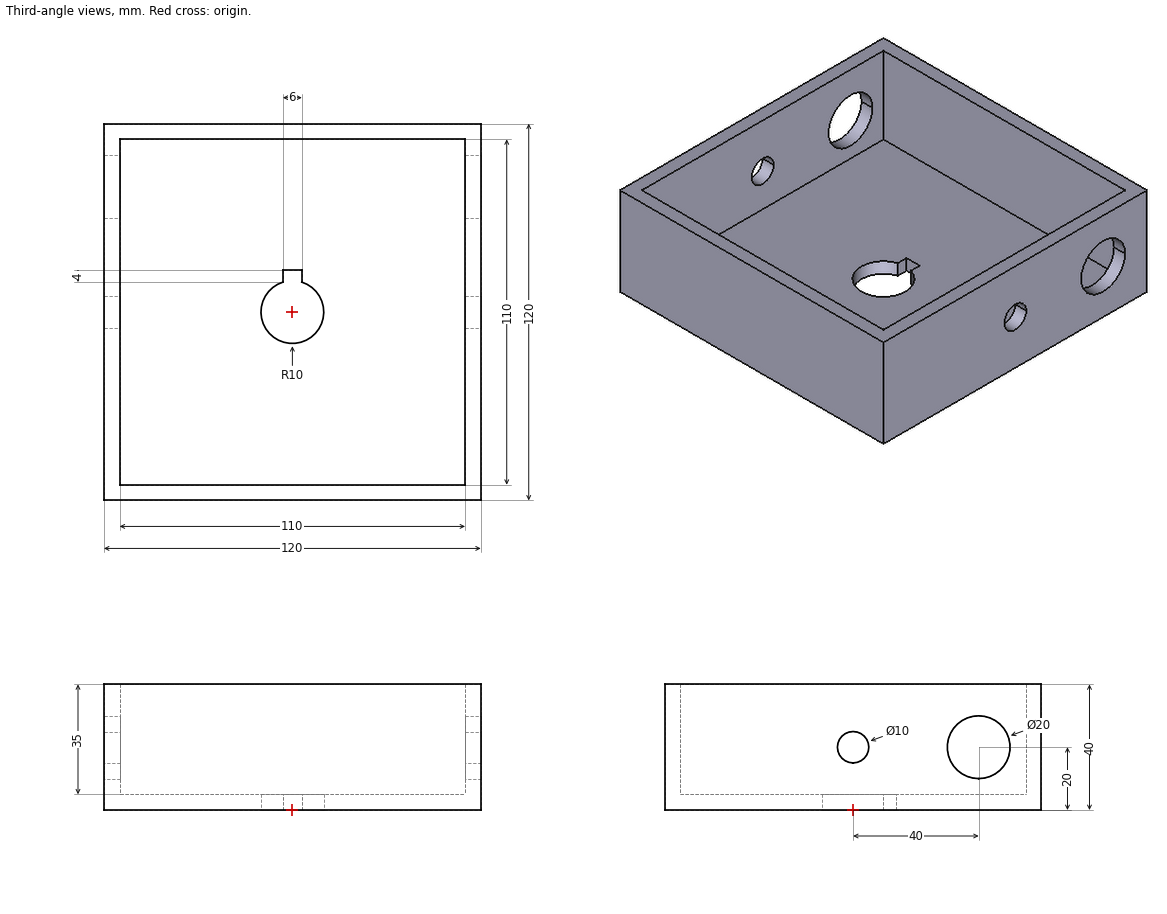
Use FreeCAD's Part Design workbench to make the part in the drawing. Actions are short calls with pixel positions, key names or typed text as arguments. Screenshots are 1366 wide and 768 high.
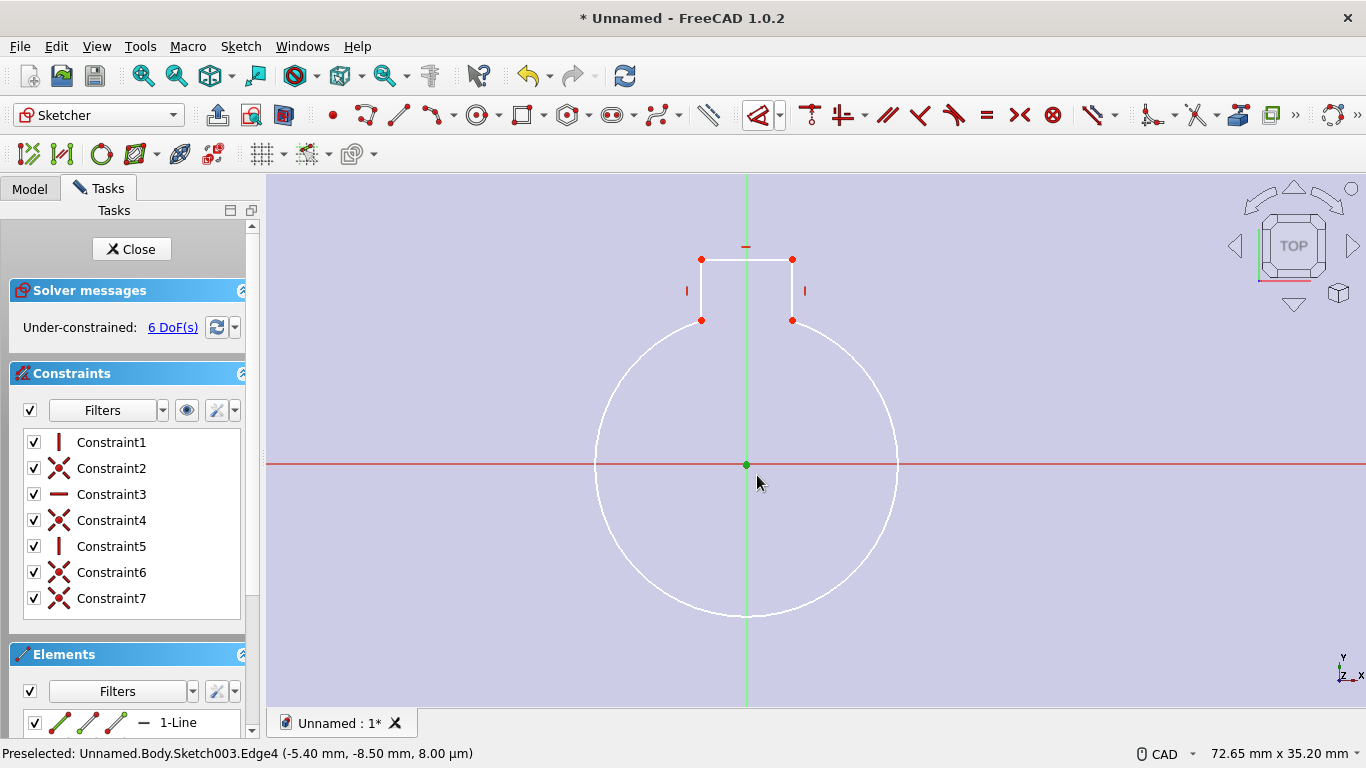
key(c)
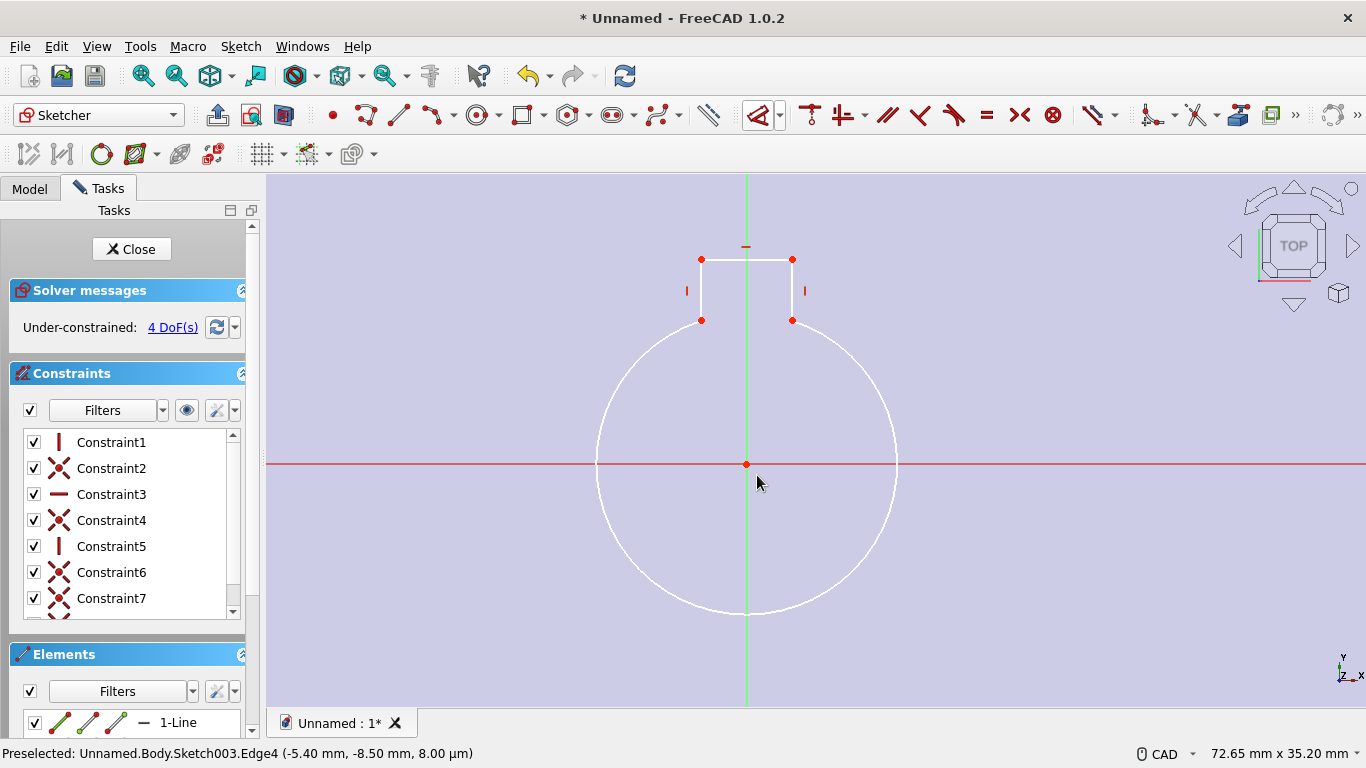
click(611, 528)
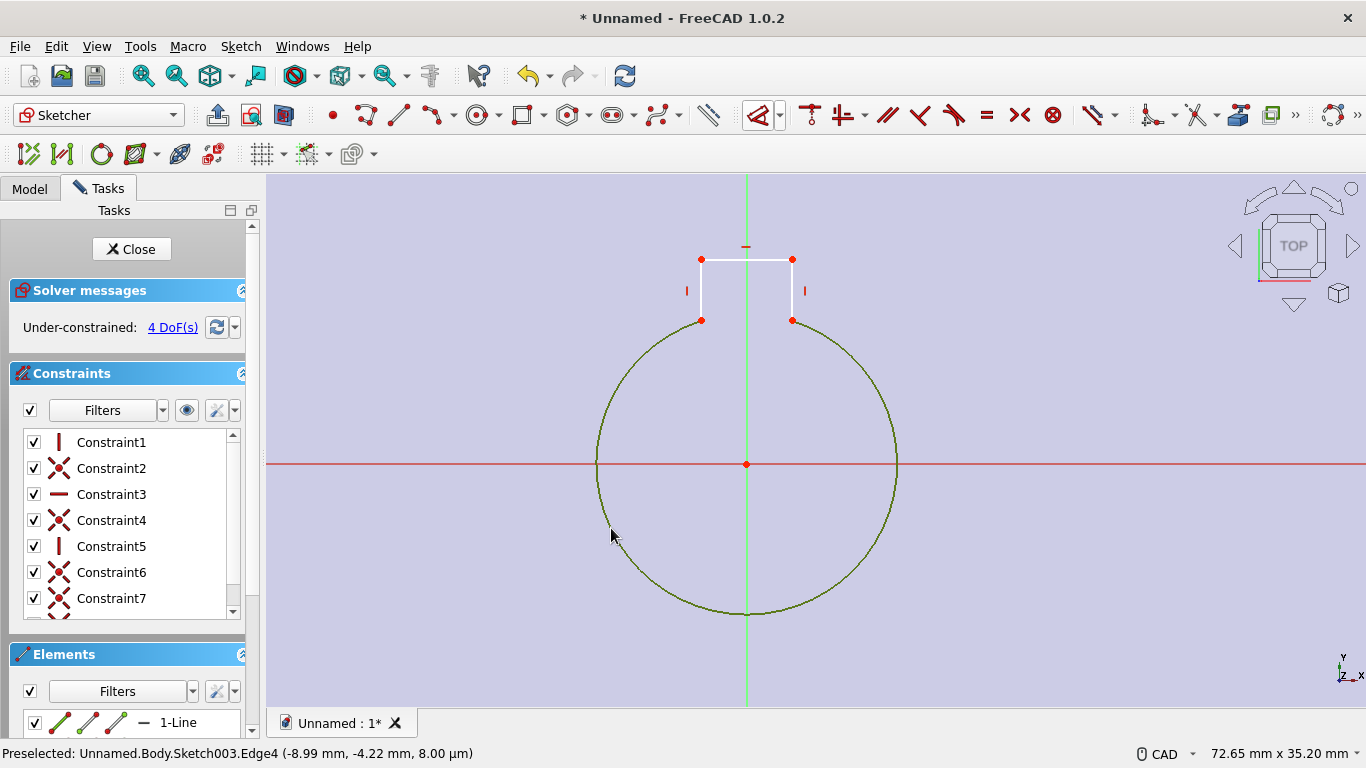
key(k)
key(r)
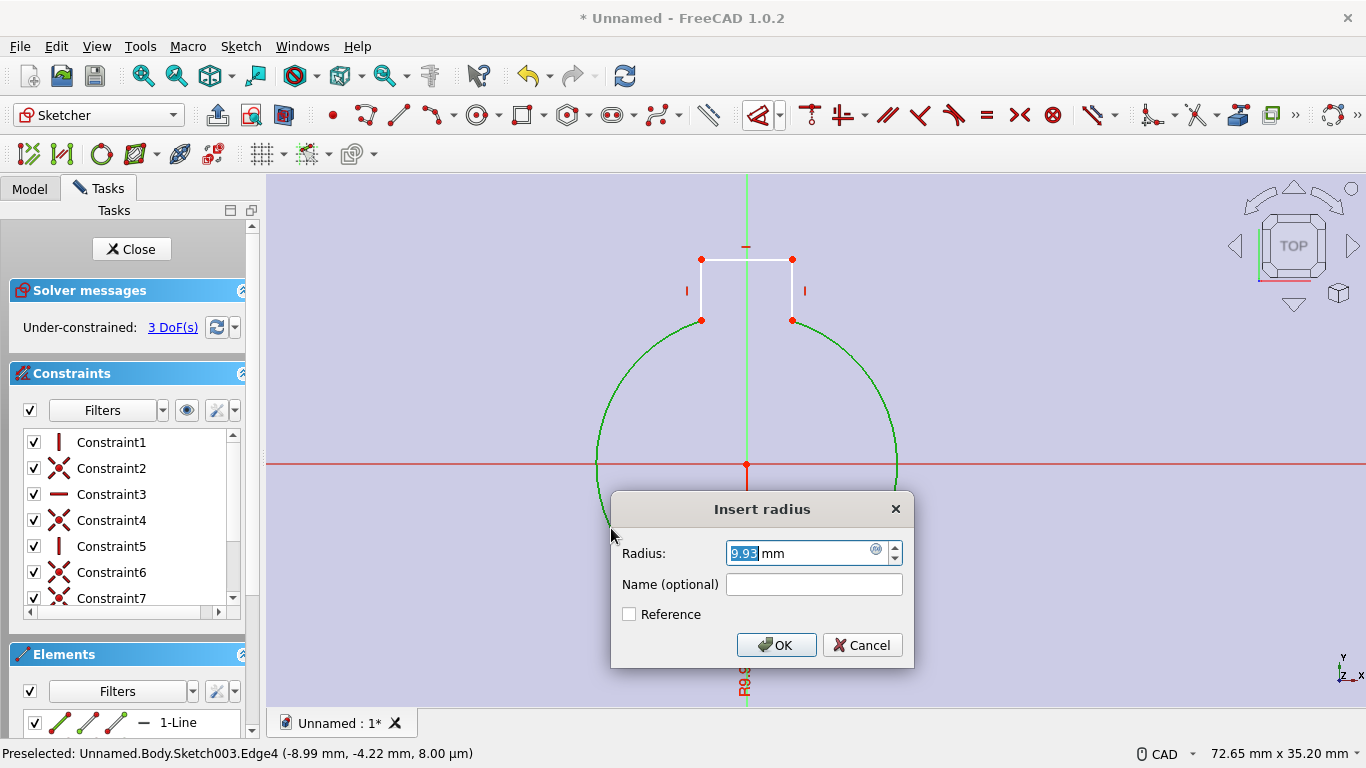
text(10)
key(Return)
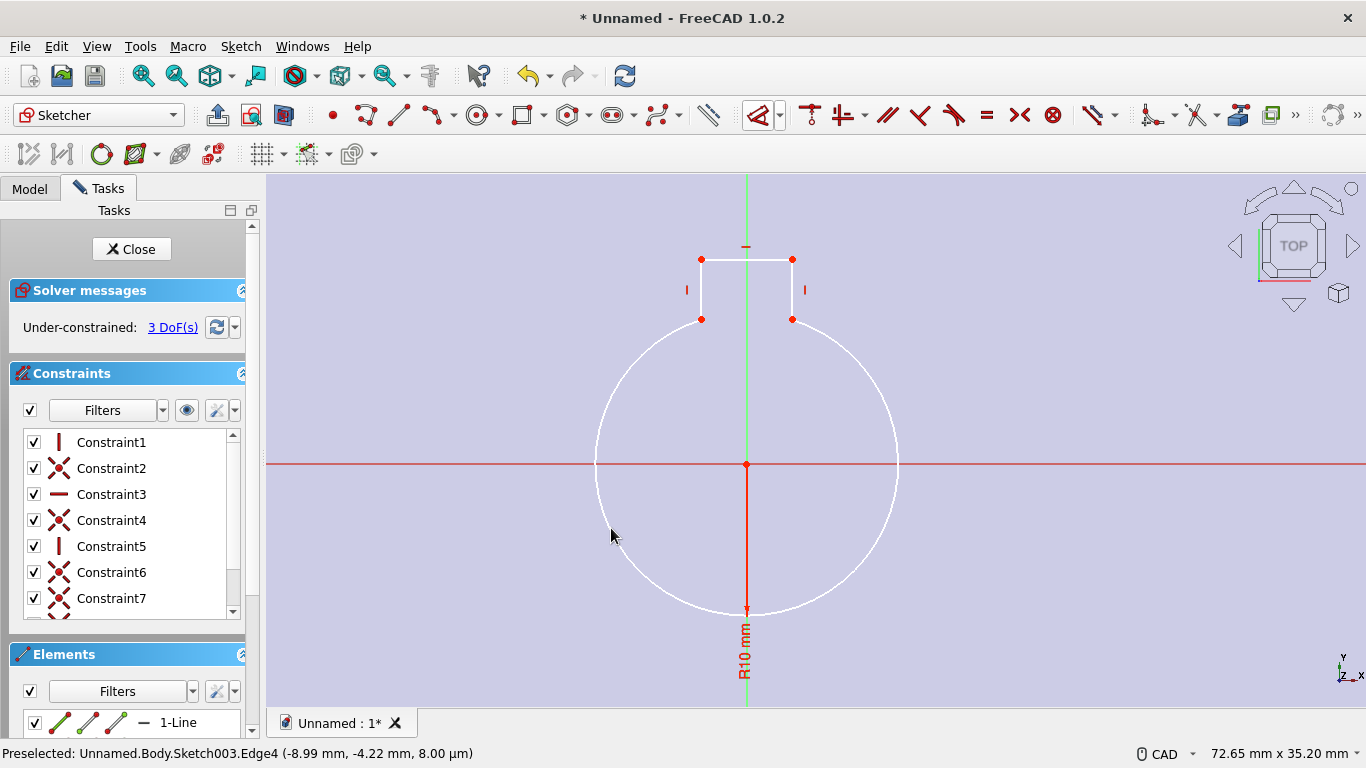
click(701, 302)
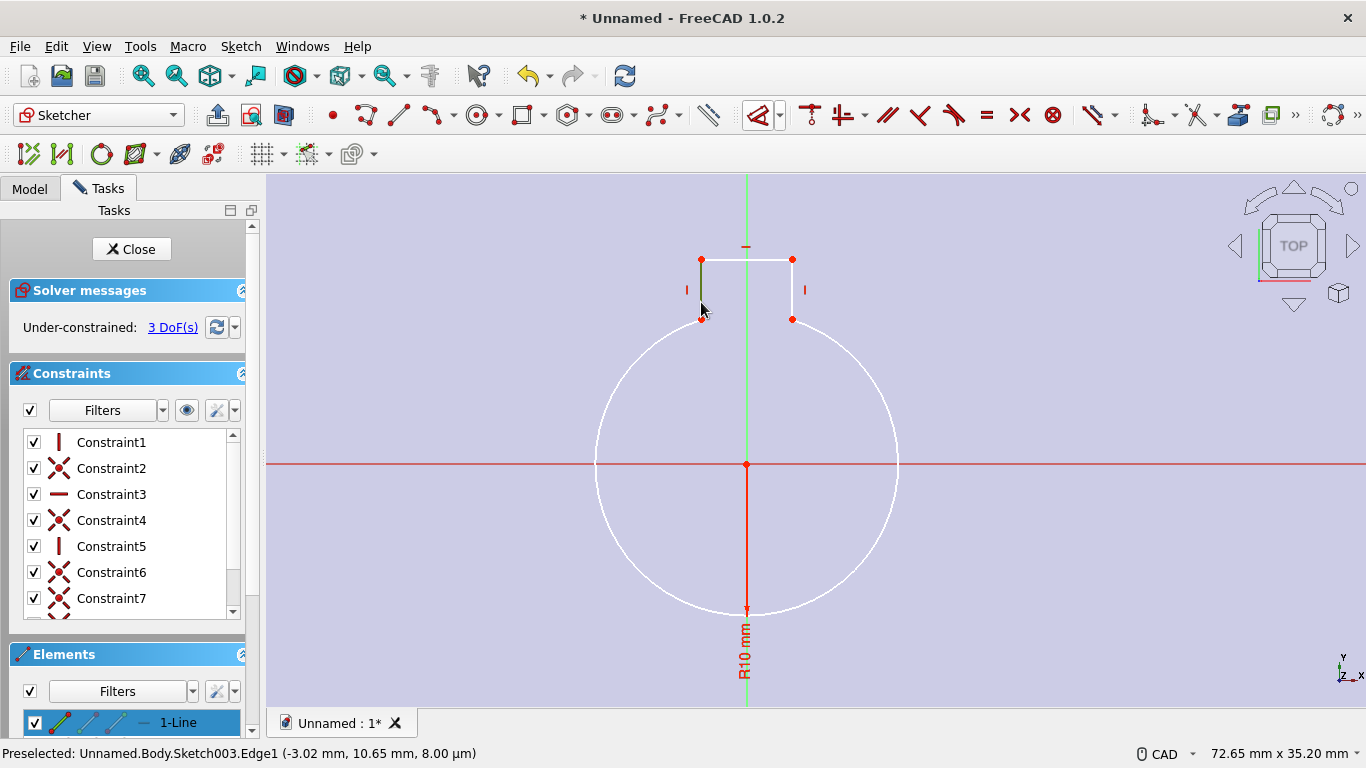
key(i)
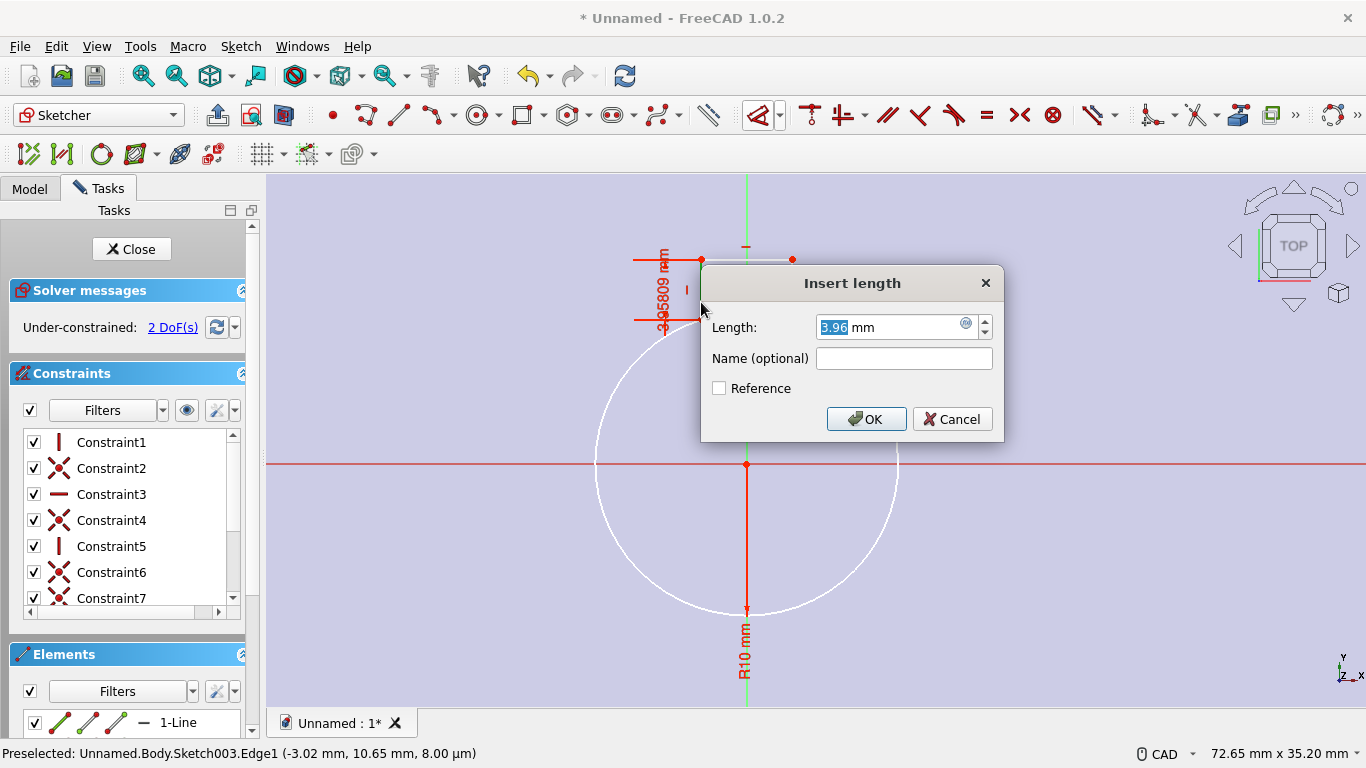
text(4)
key(Return)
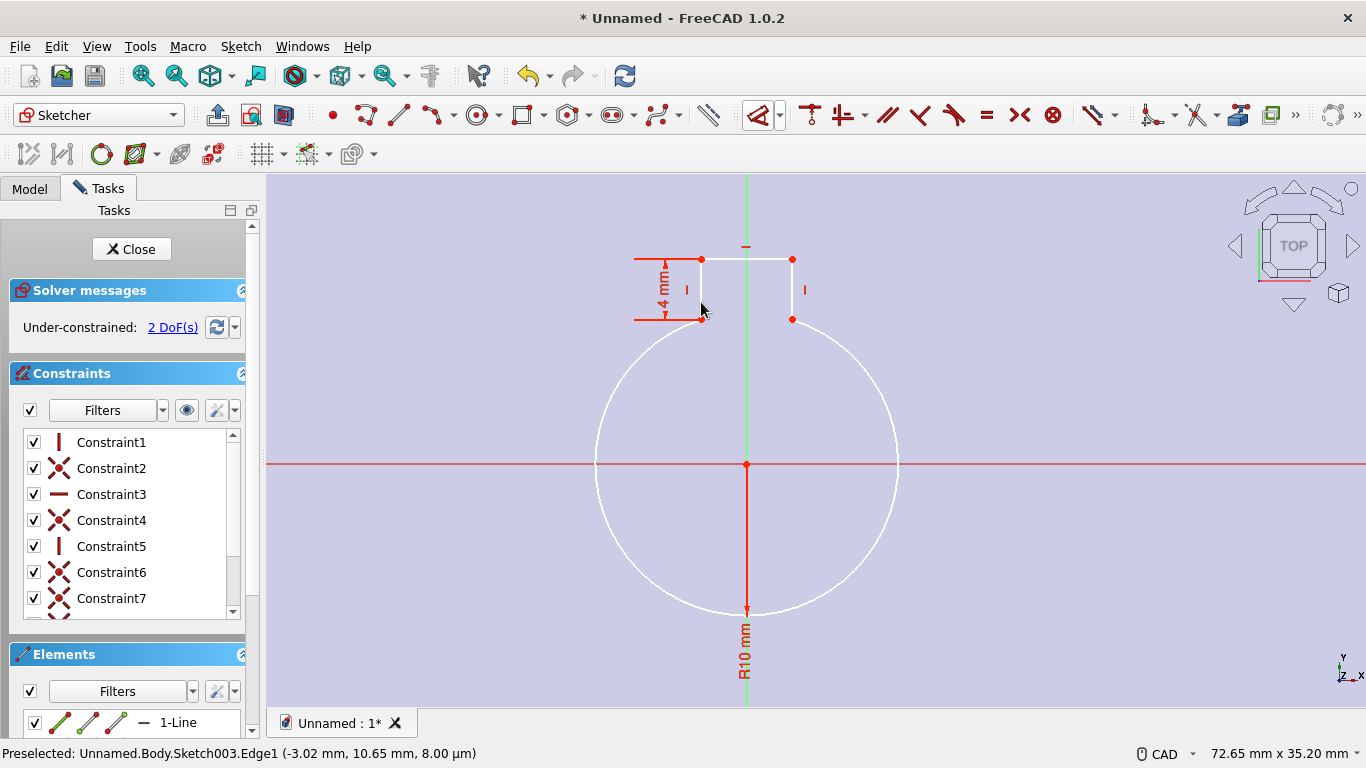
click(728, 259)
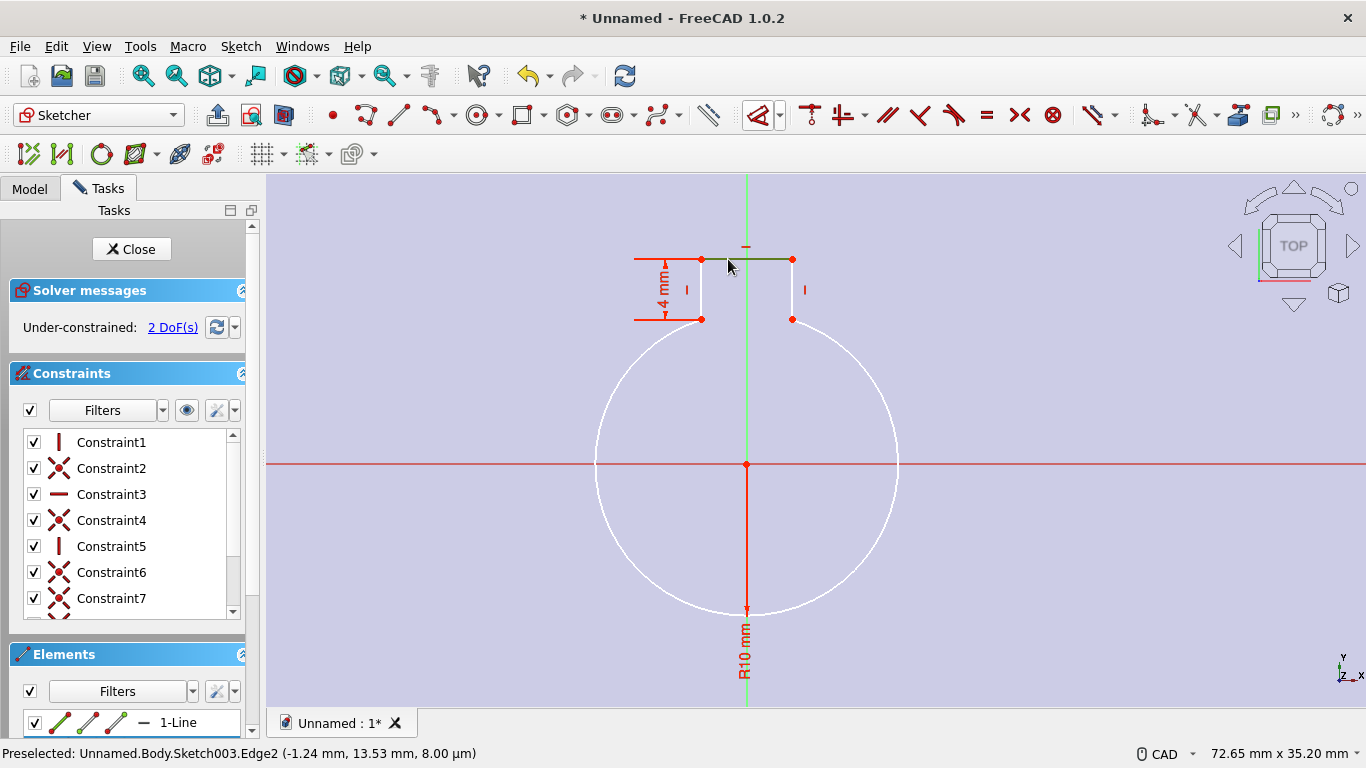
key(l)